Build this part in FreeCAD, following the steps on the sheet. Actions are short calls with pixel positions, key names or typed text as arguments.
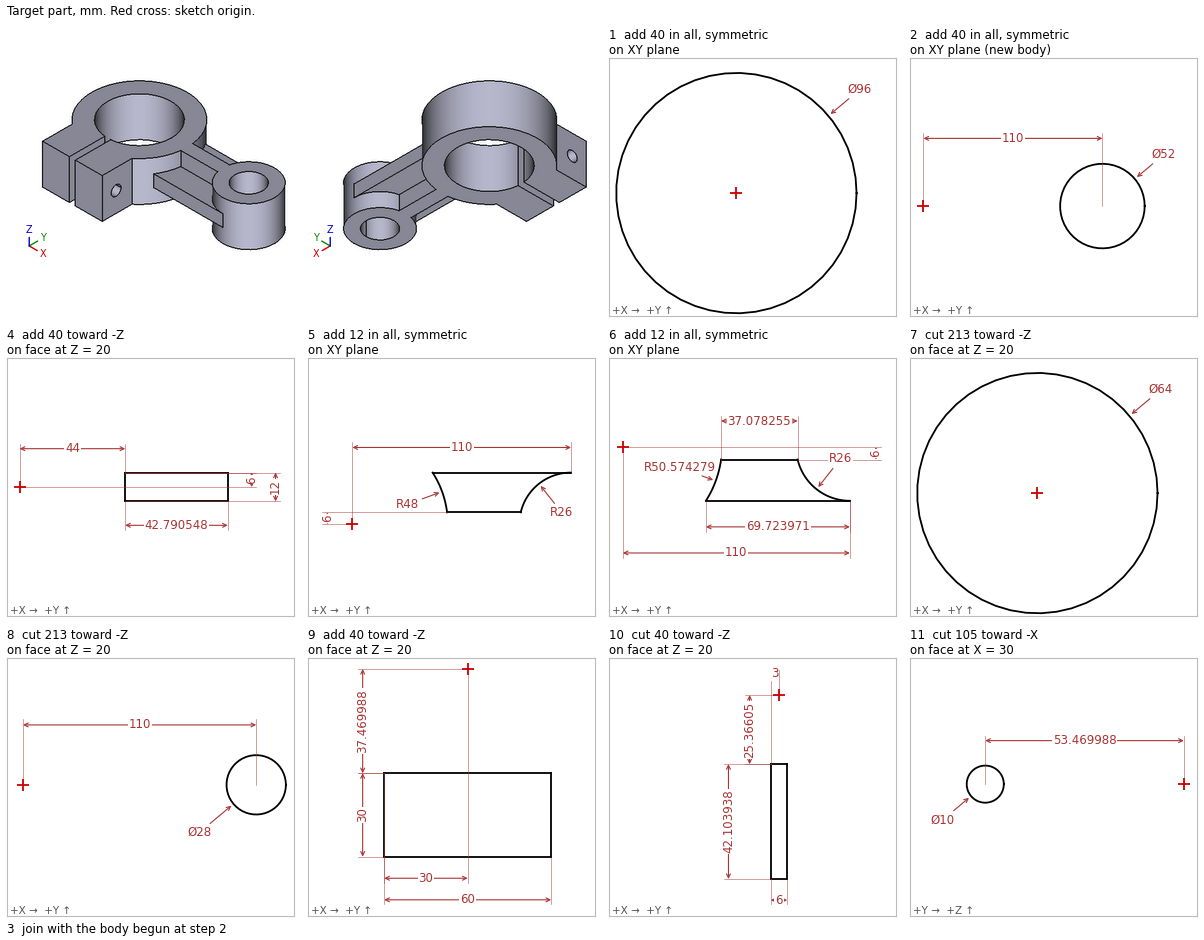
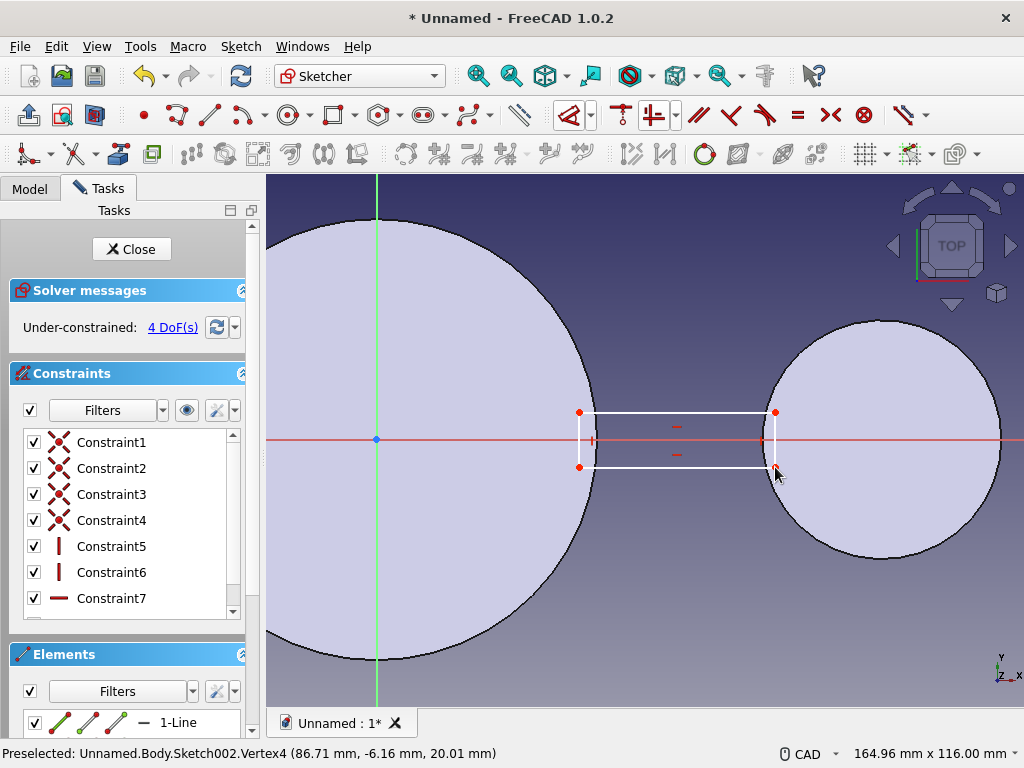
scroll(579, 430, up, 2)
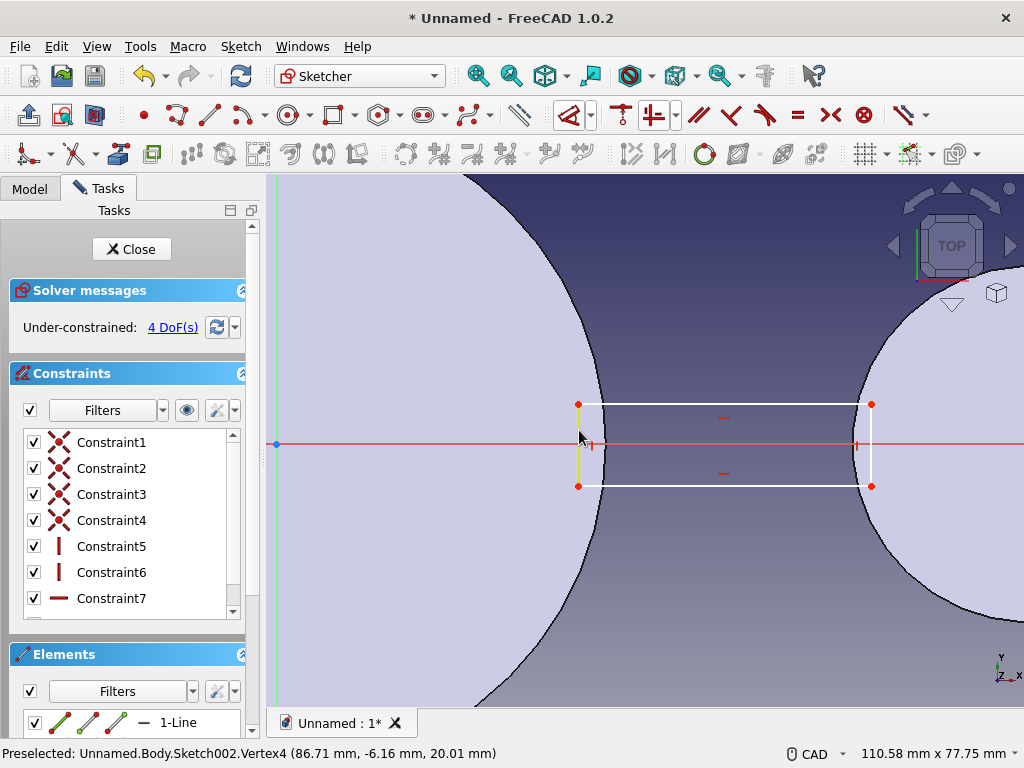
click(579, 429)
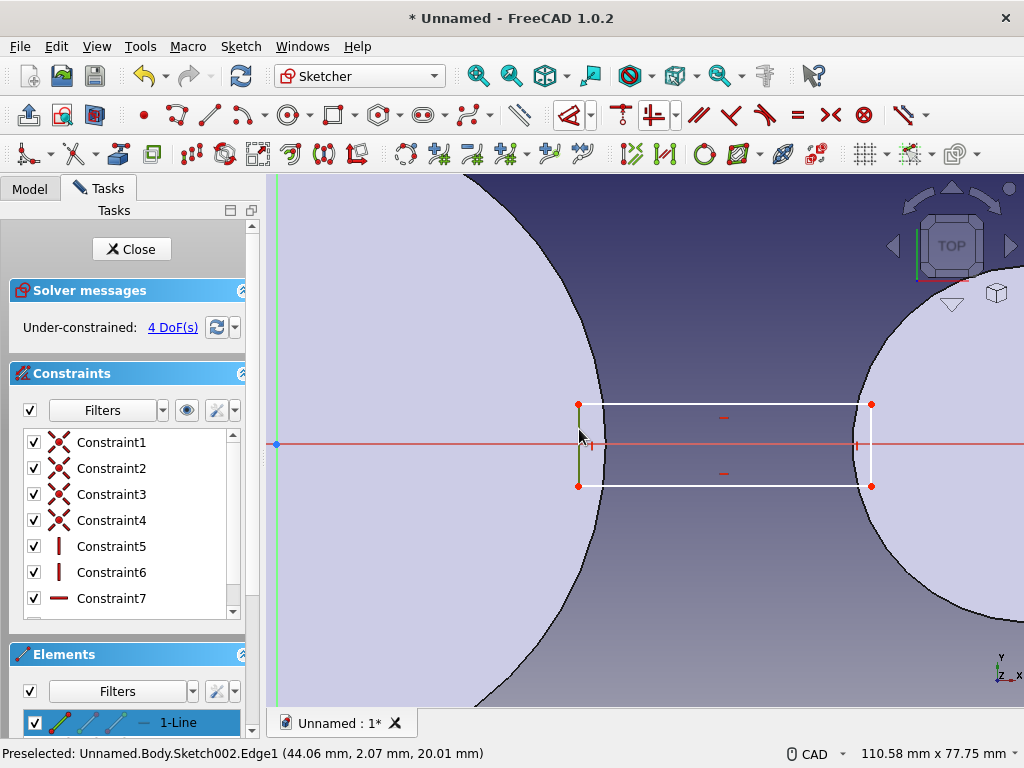
click(590, 116)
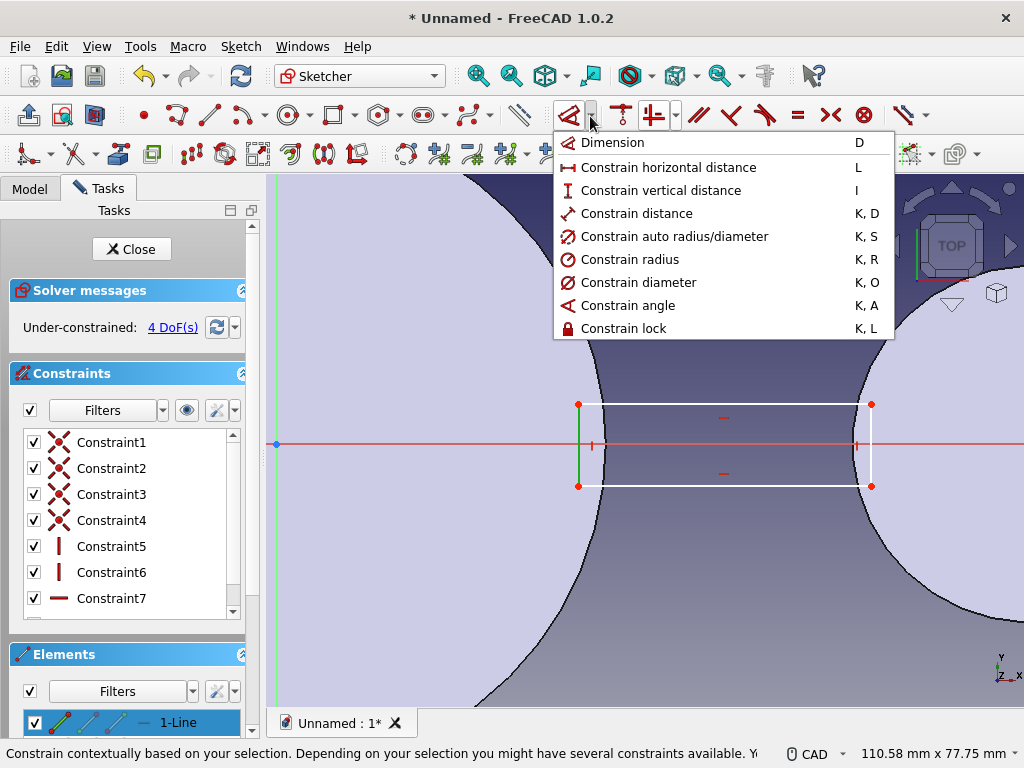
click(724, 190)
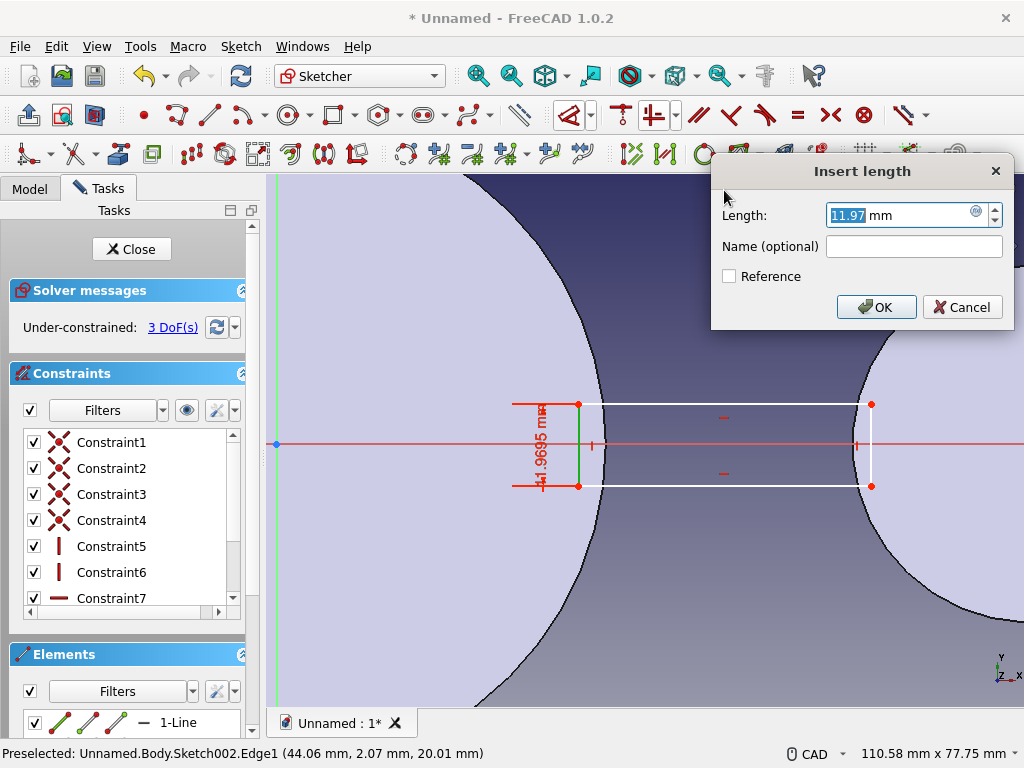
text(12)
key(Return)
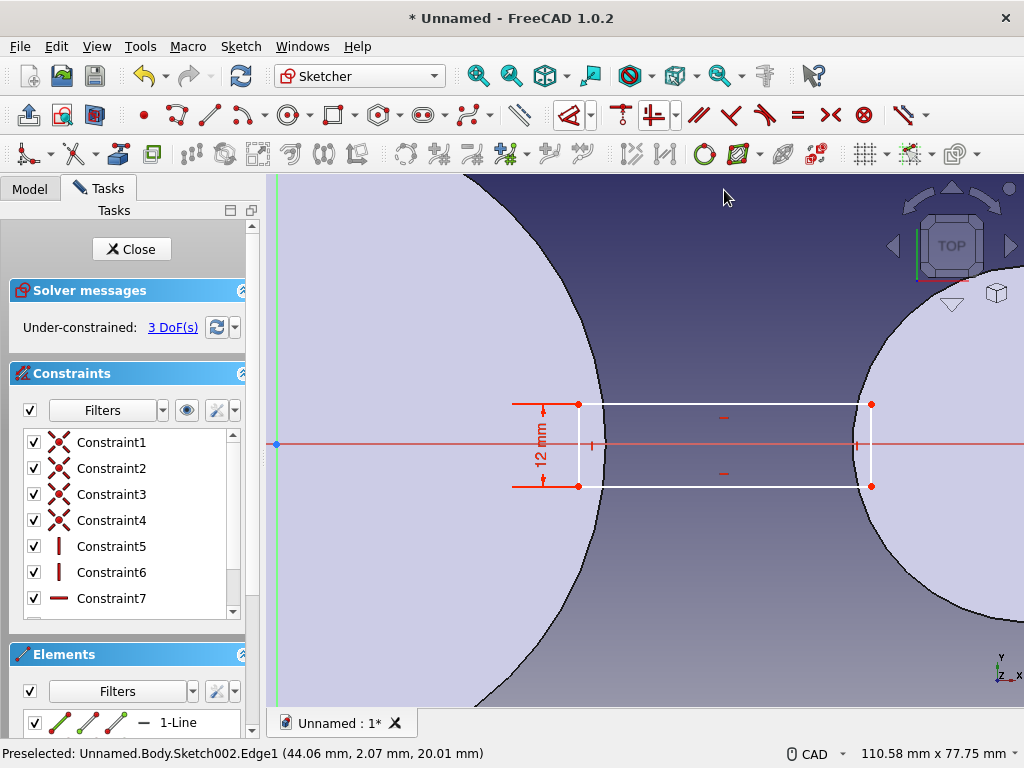
click(579, 404)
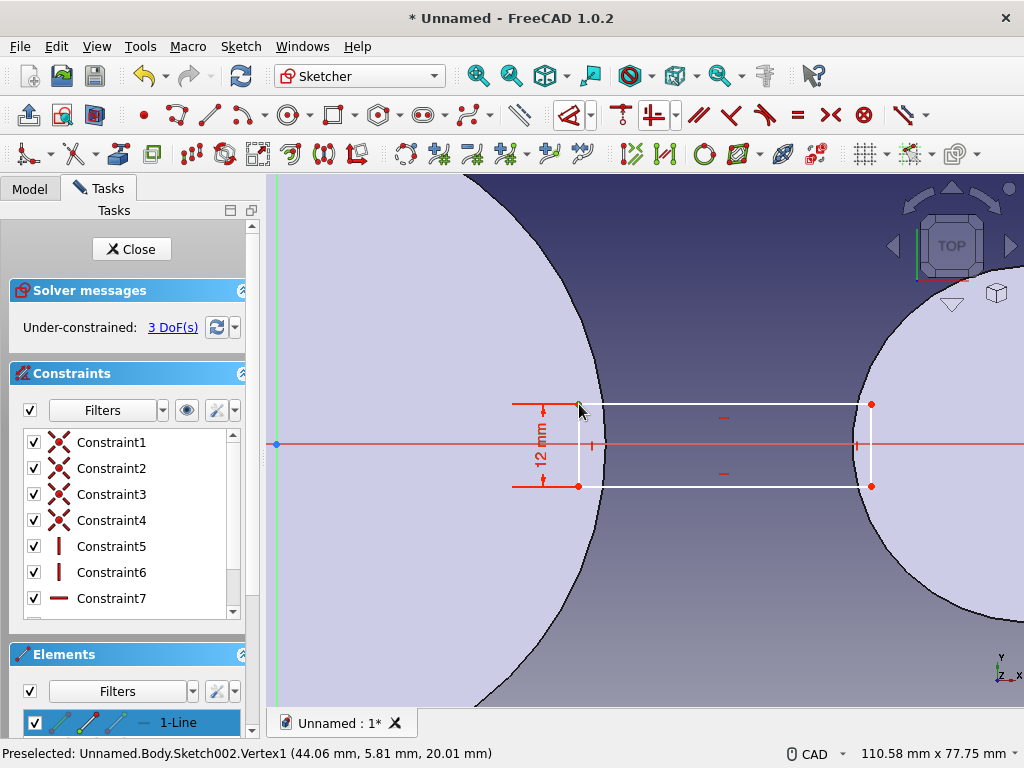
key(i)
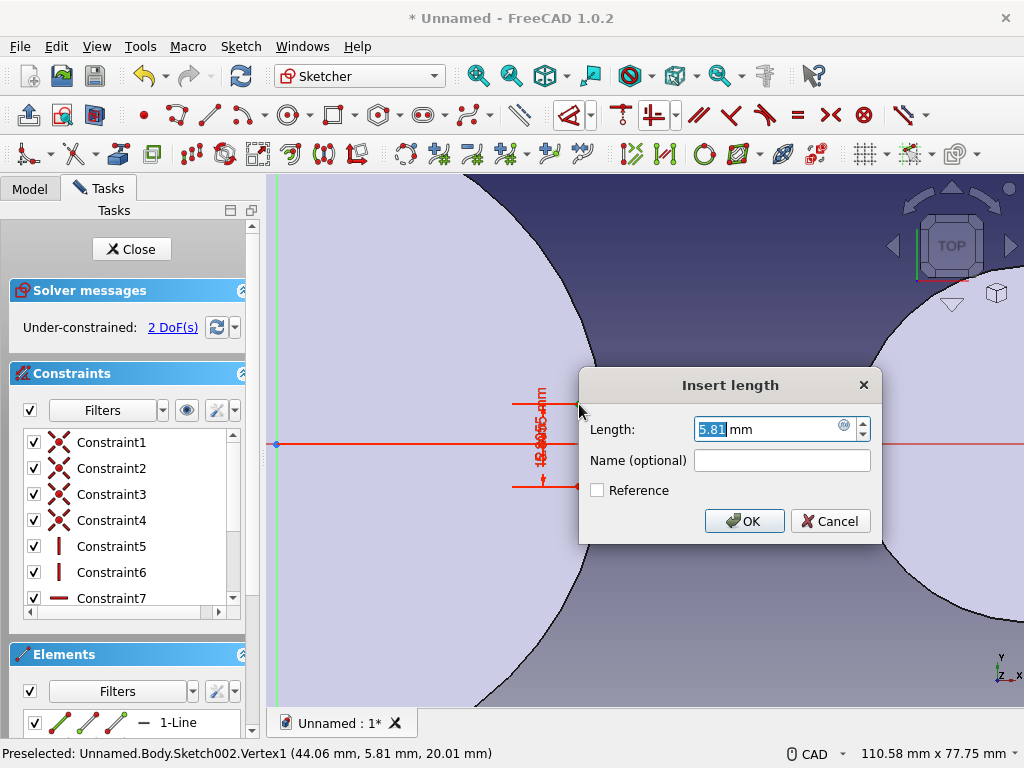
text(6)
key(Return)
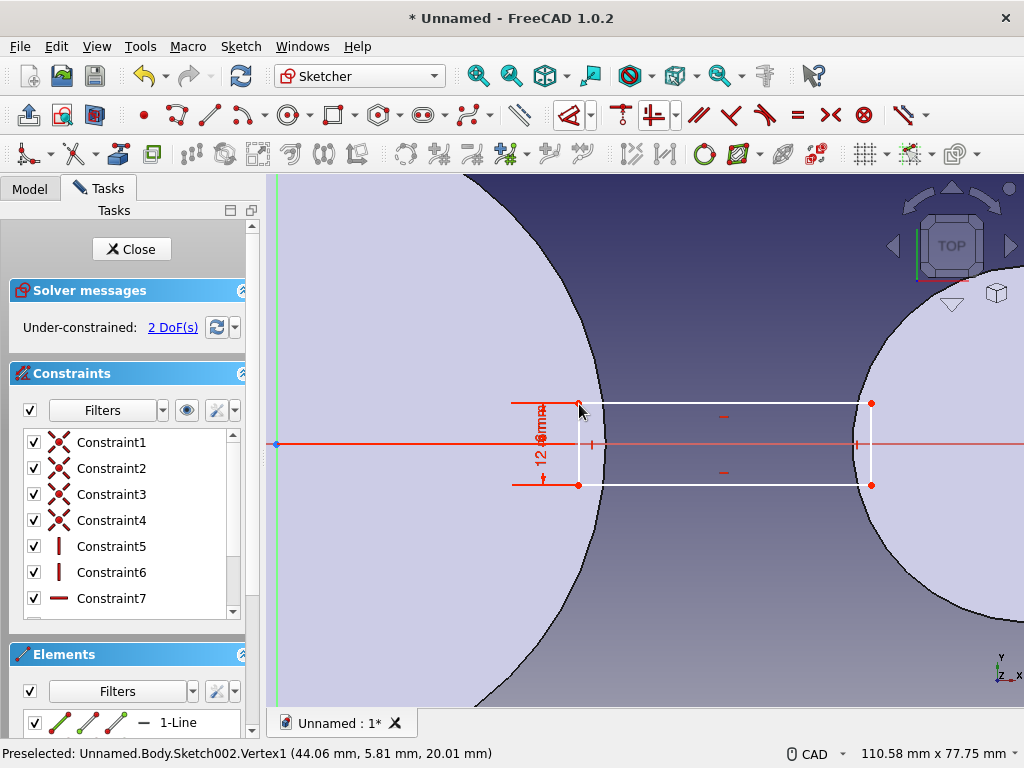
click(579, 403)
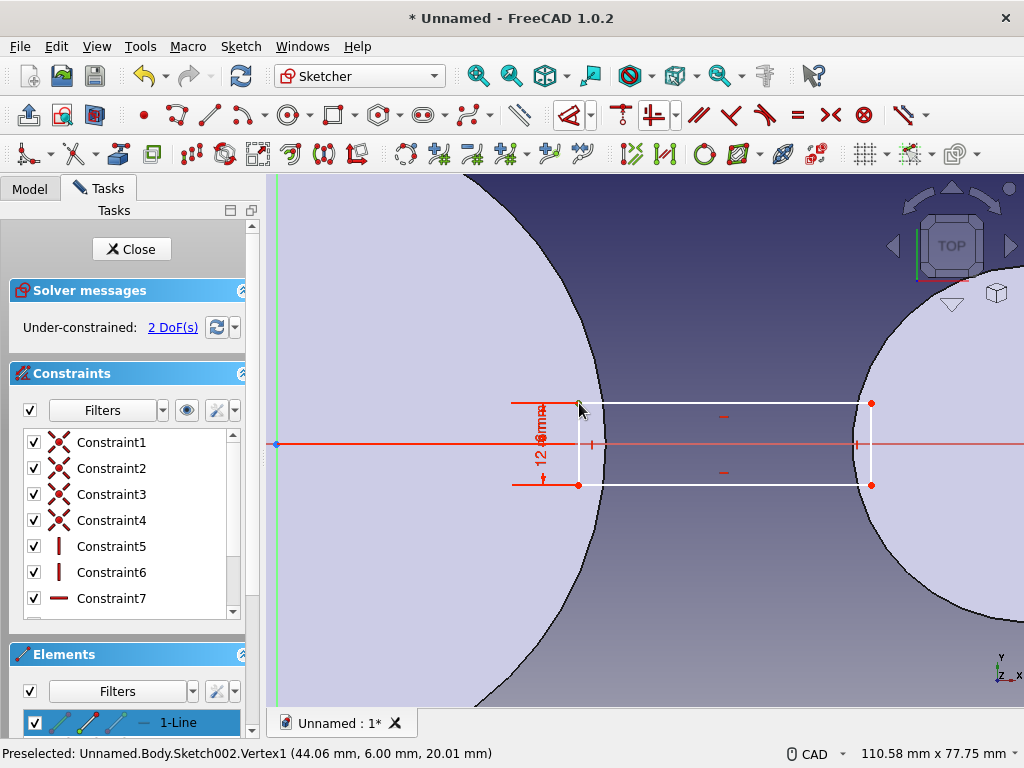
key(l)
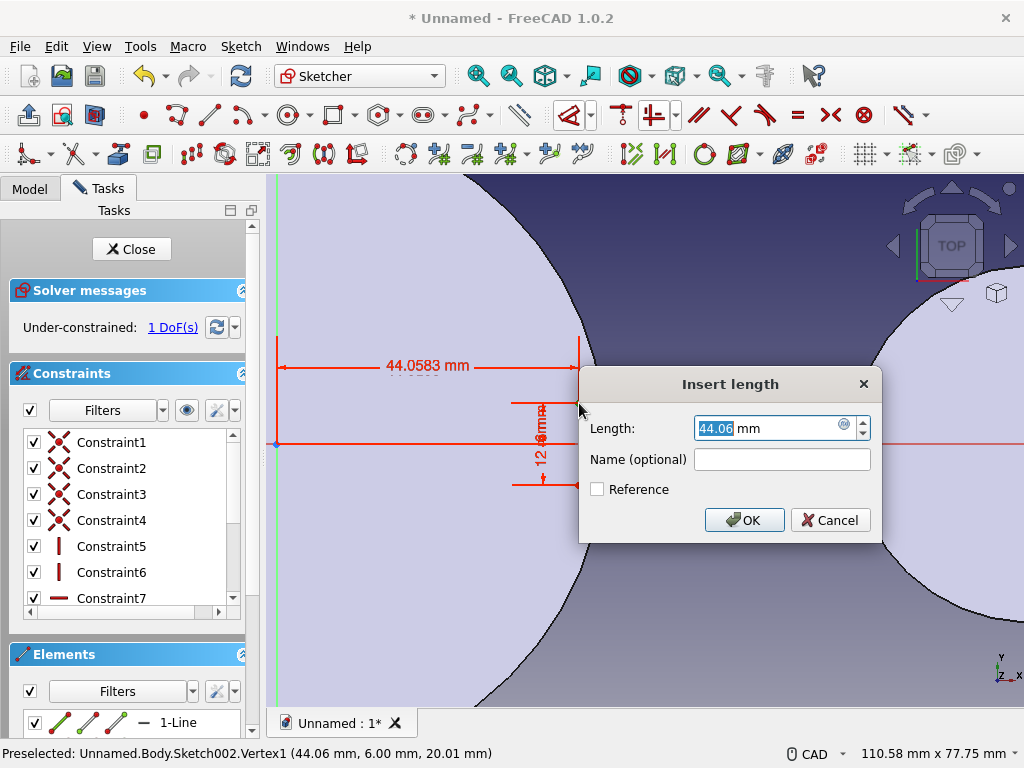
text(44)
key(Return)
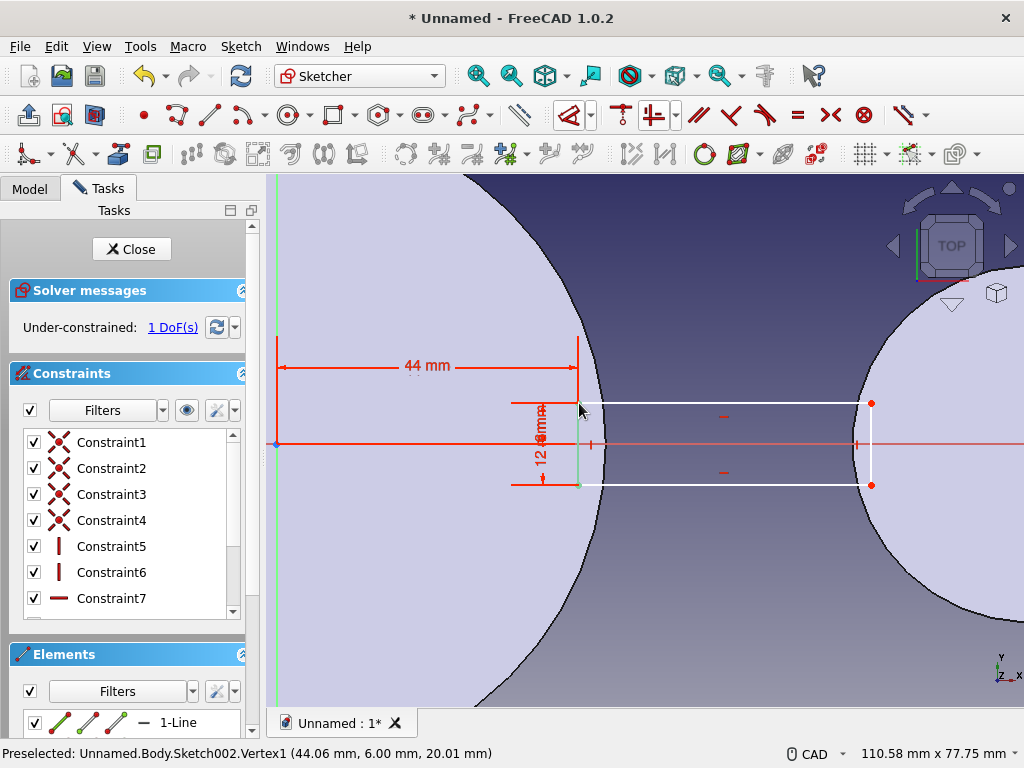
click(666, 485)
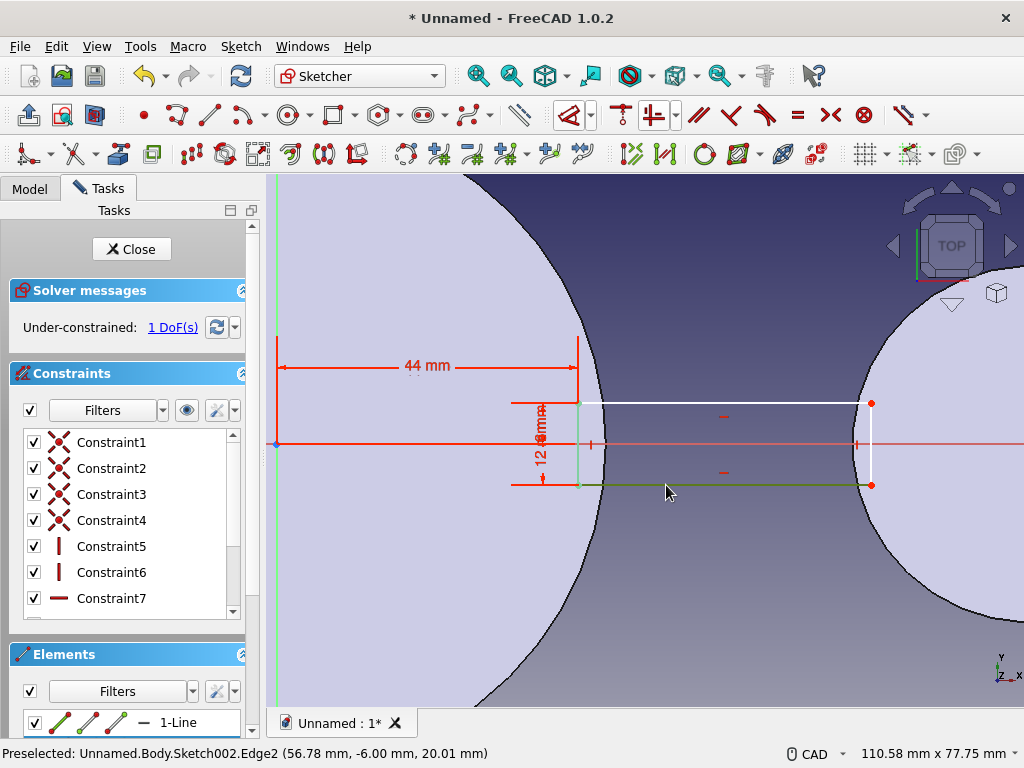
click(590, 116)